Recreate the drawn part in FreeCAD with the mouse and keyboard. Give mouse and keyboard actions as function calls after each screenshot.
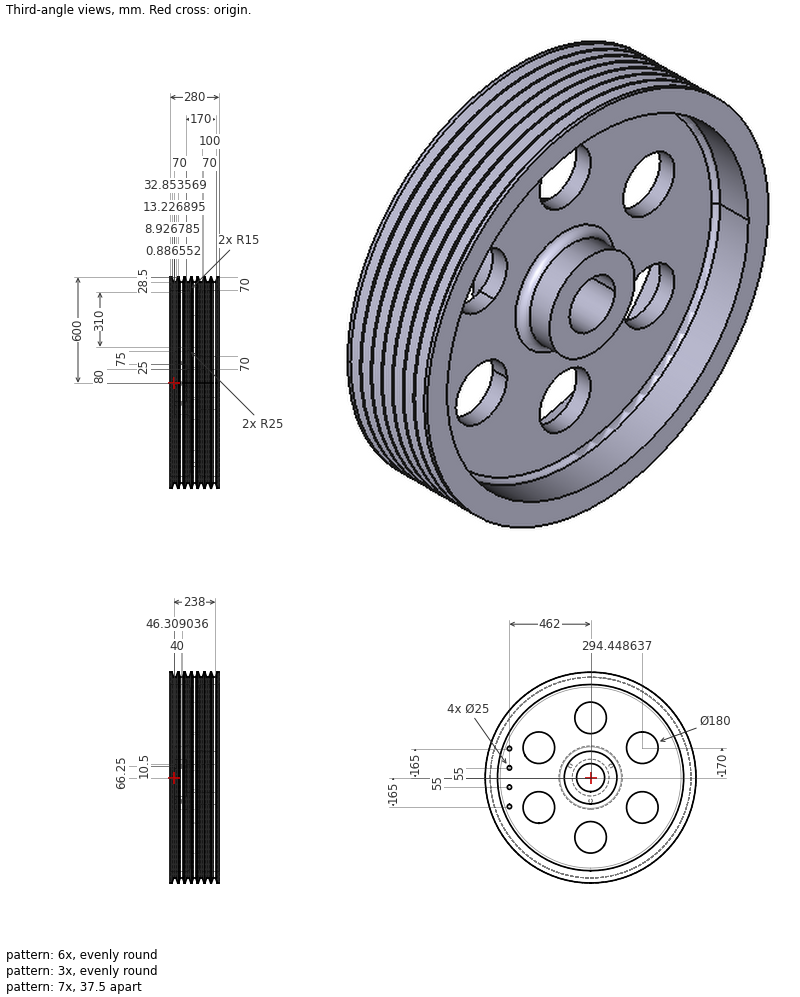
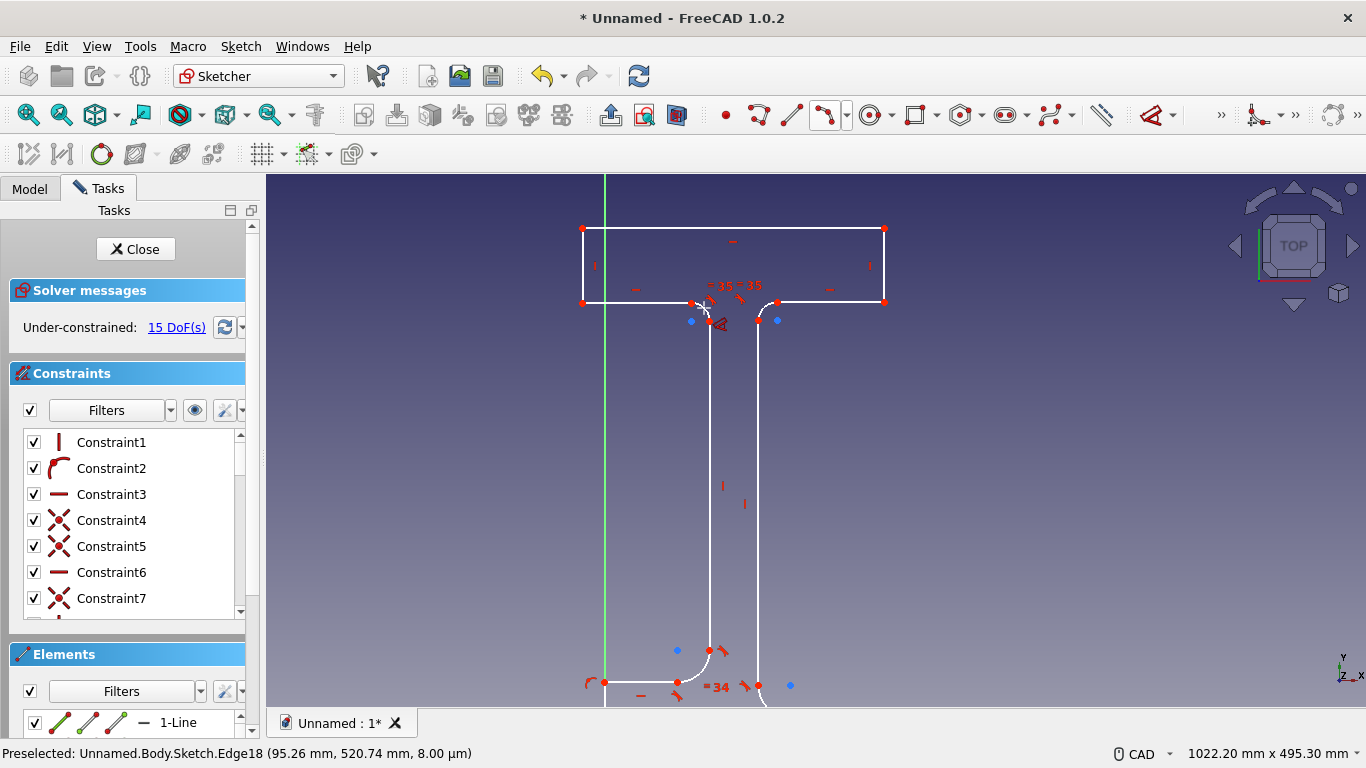
scroll(692, 679, up, 2)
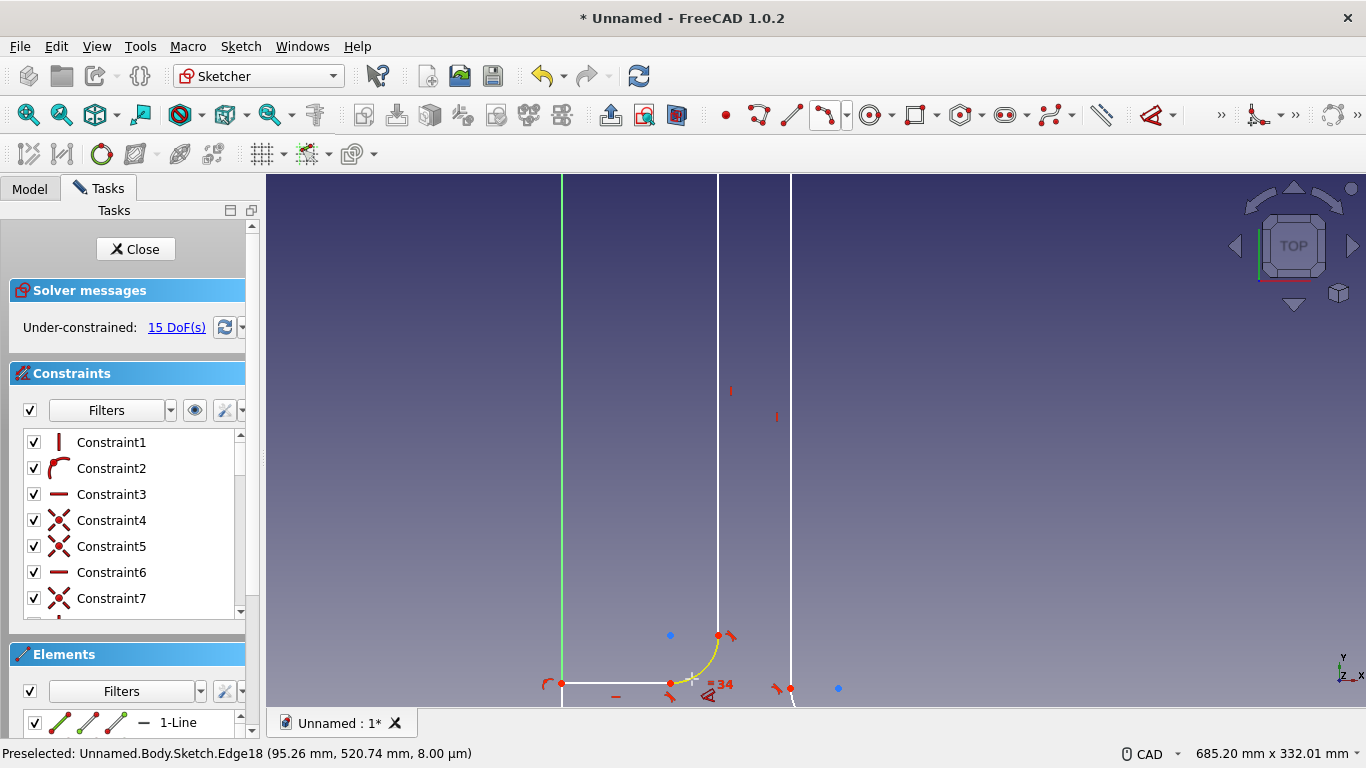
click(693, 678)
click(750, 643)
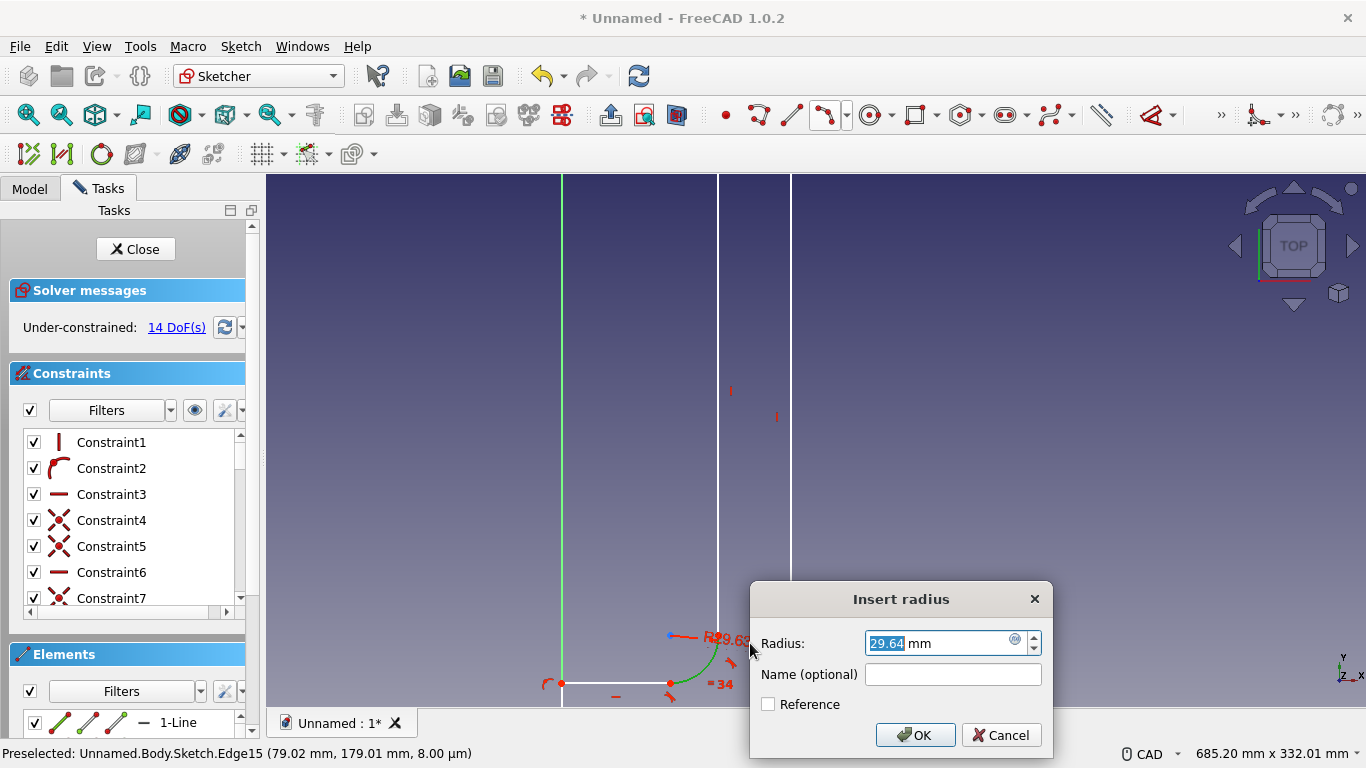
text(25)
key(Return)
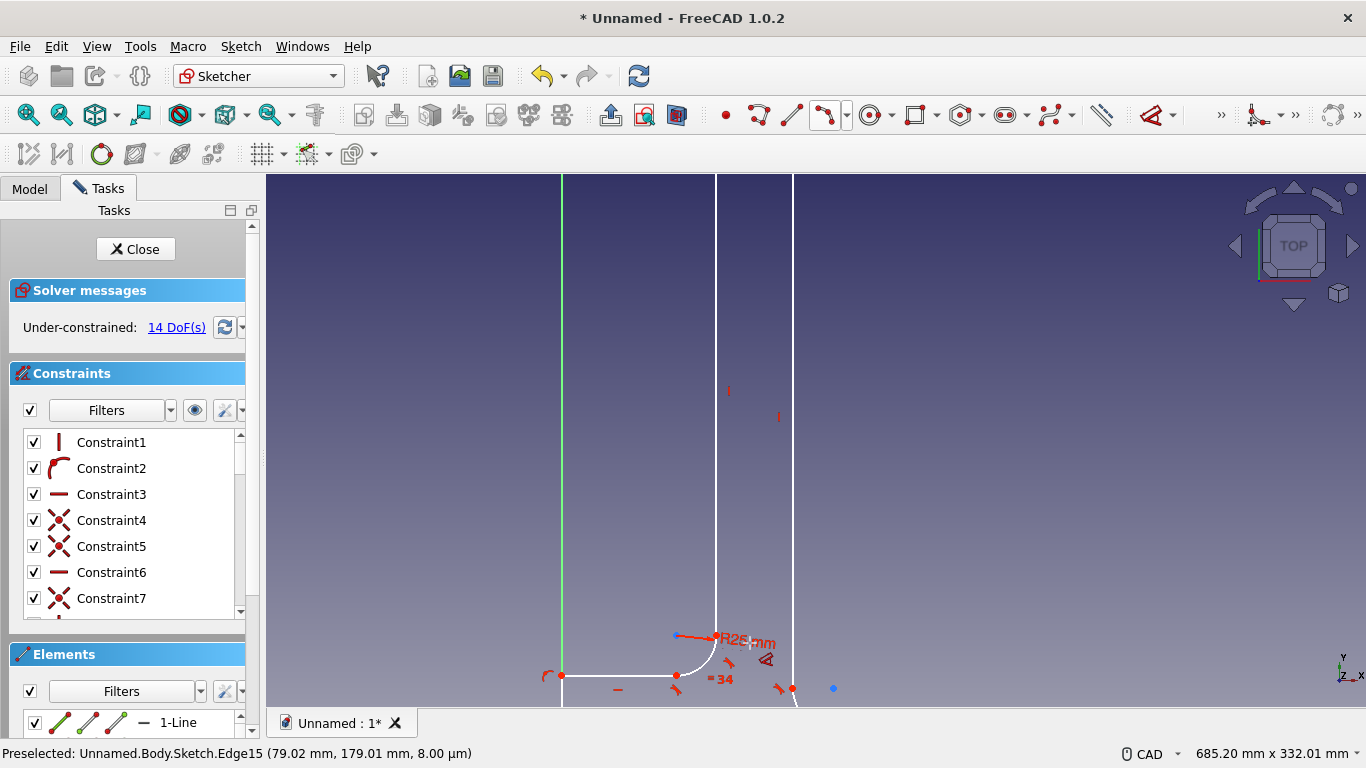
scroll(744, 414, down, 5)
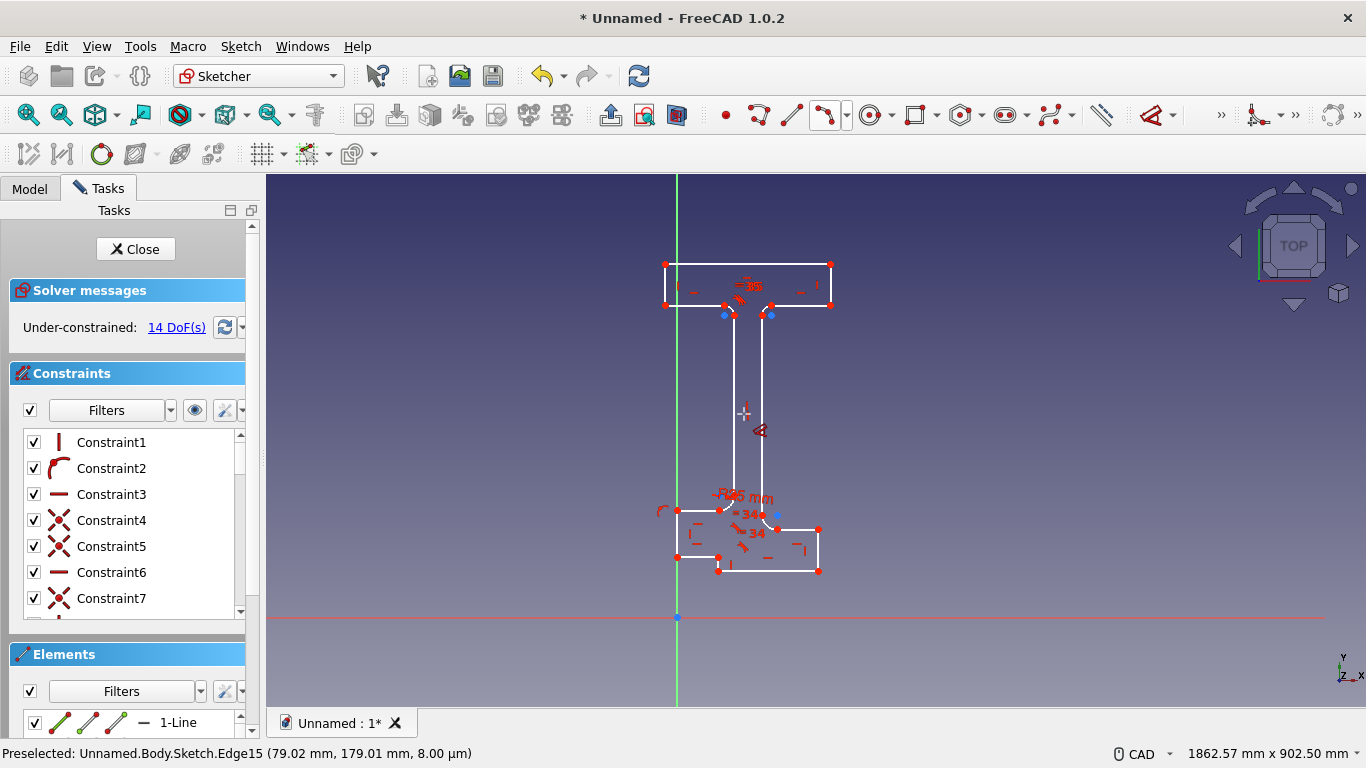
scroll(767, 307, up, 8)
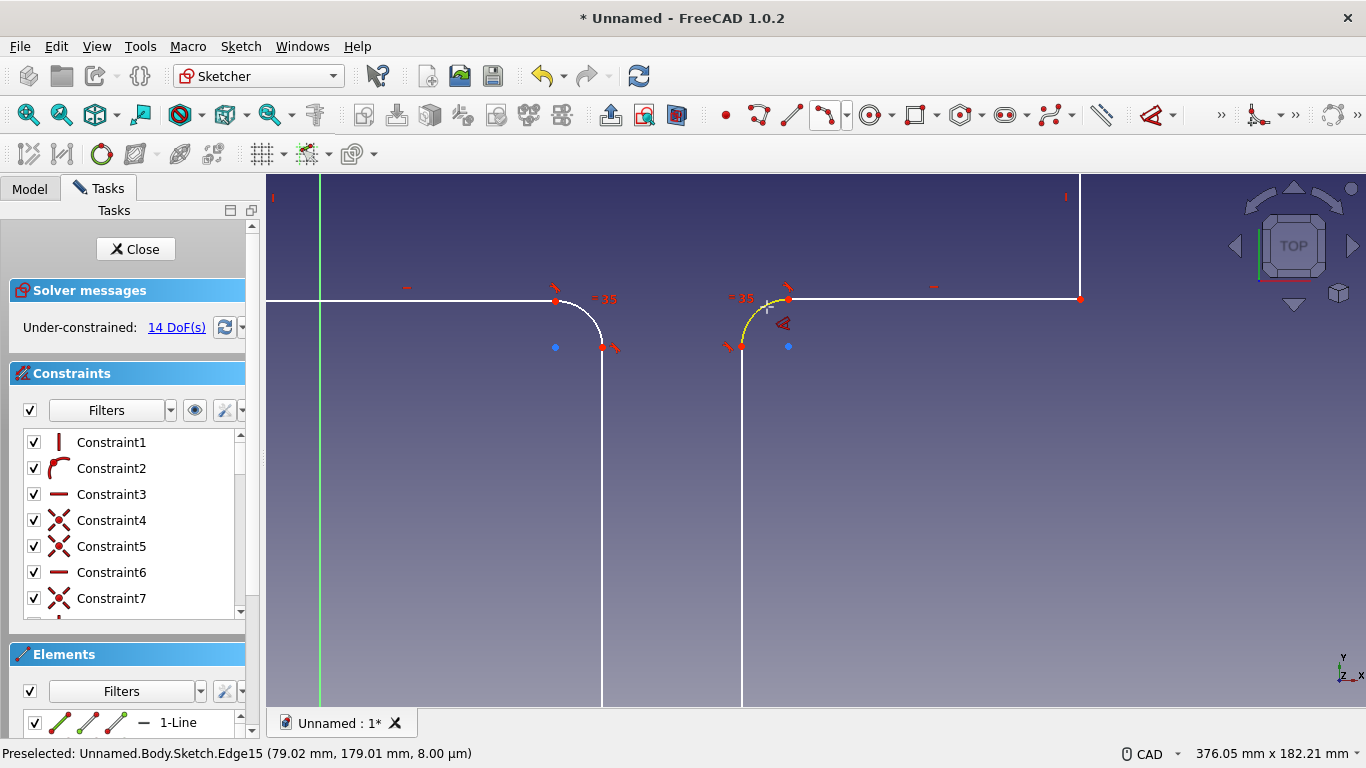
click(767, 304)
click(752, 276)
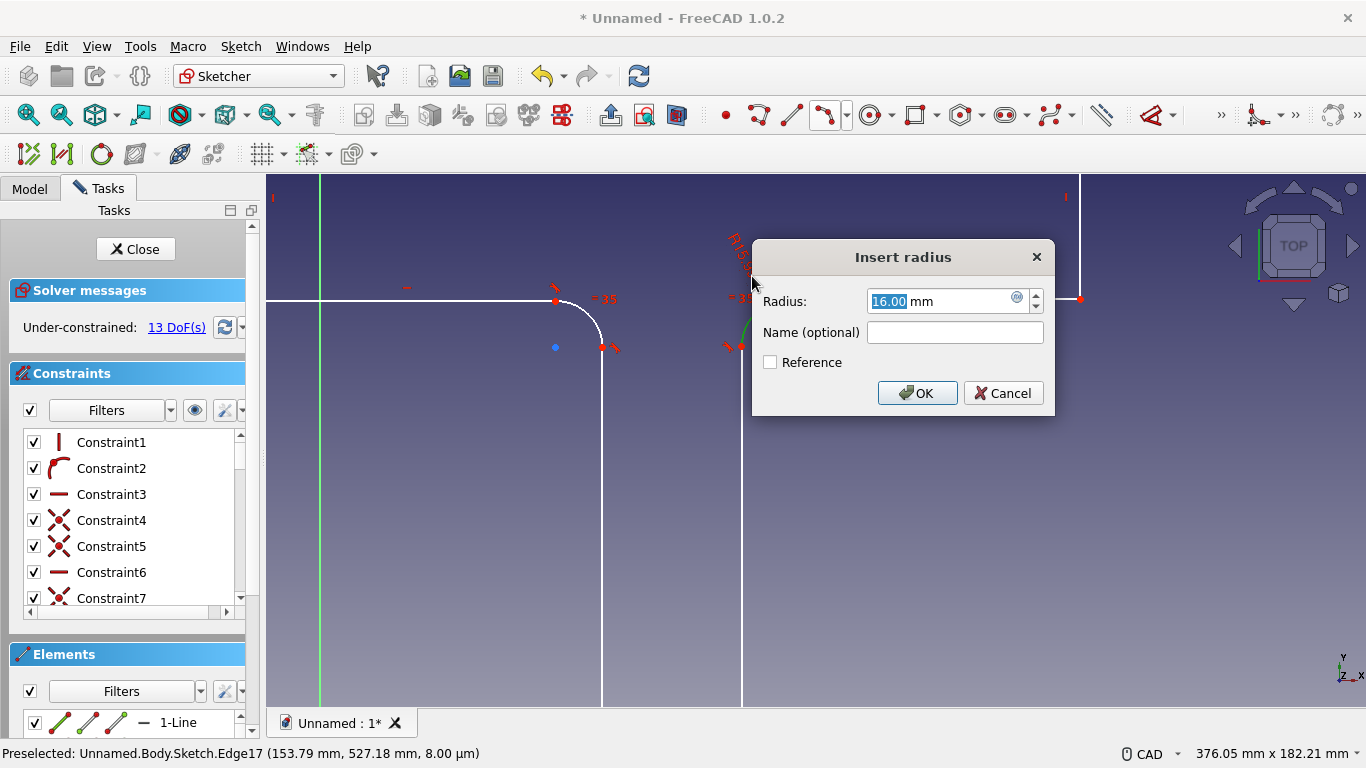
text(15)
key(Return)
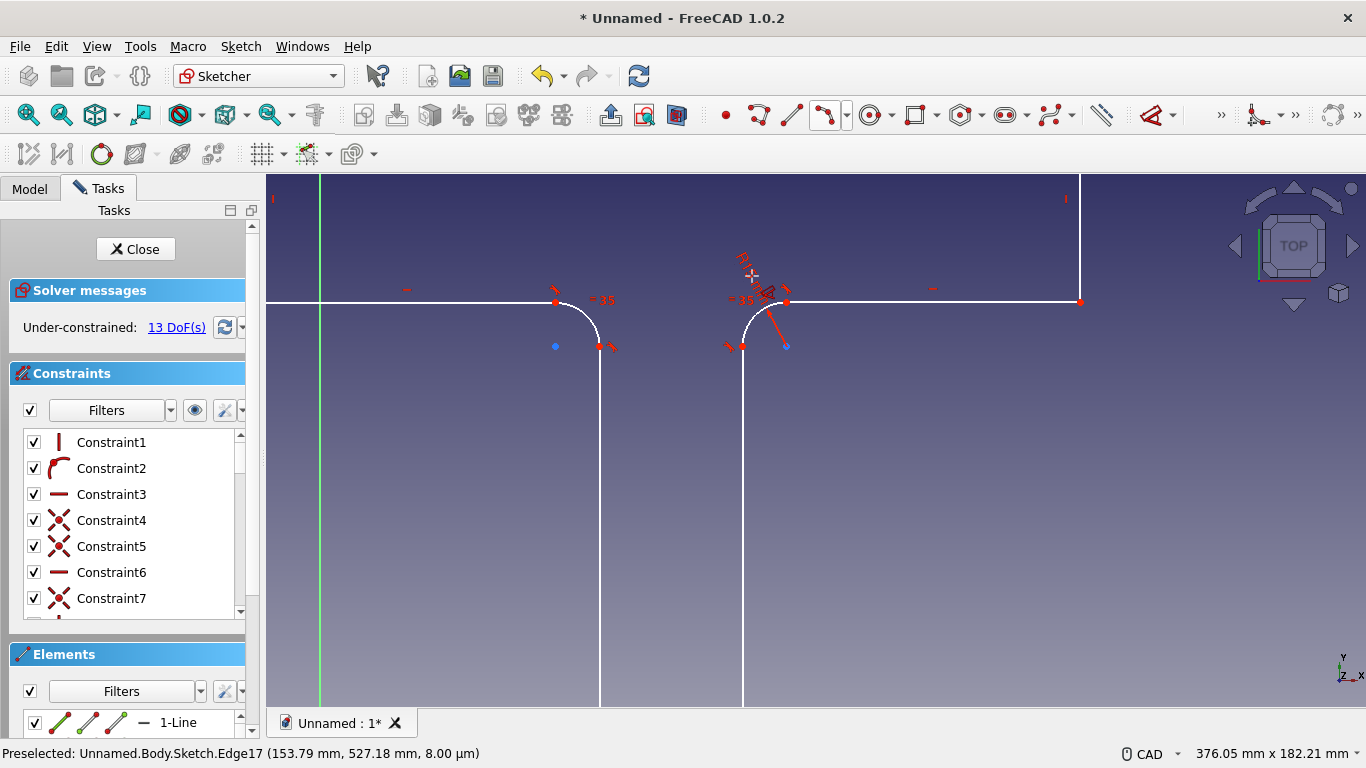
scroll(767, 307, down, 8)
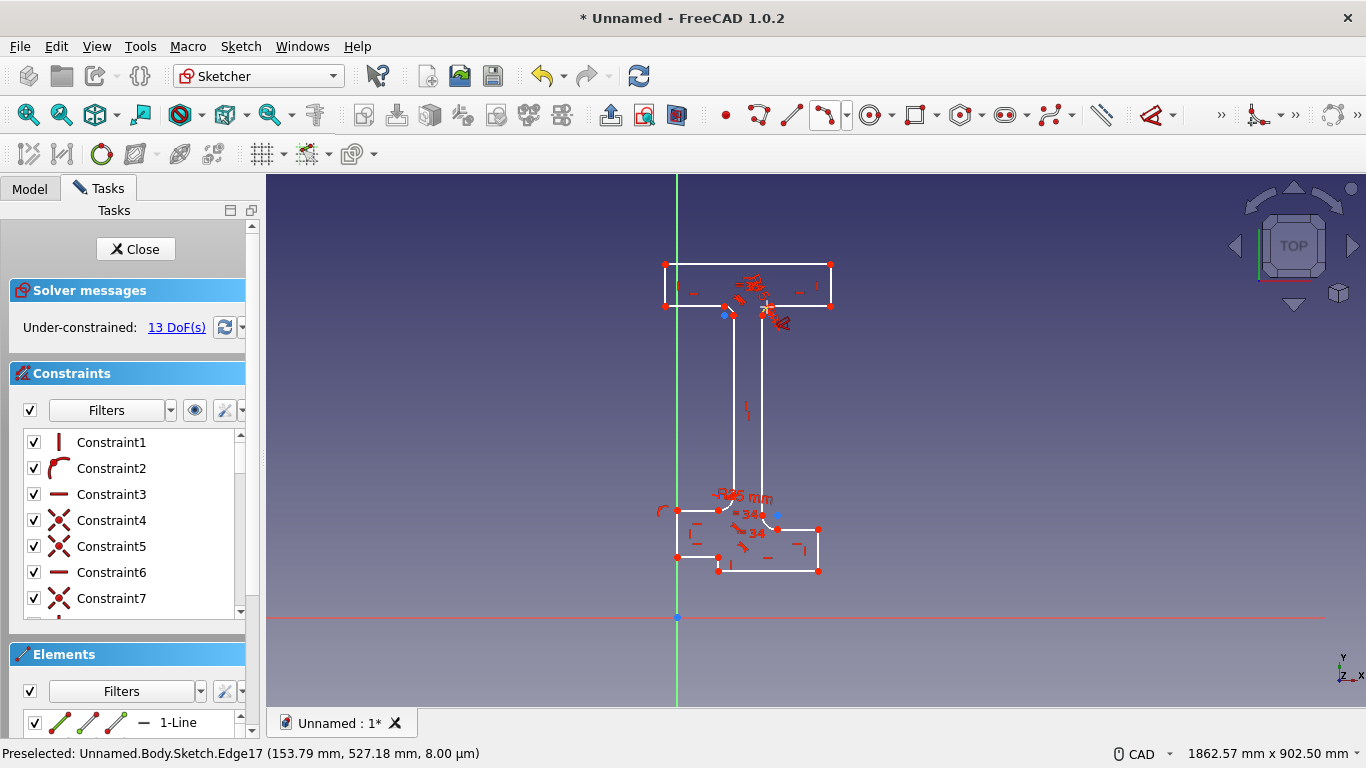
click(706, 511)
click(698, 477)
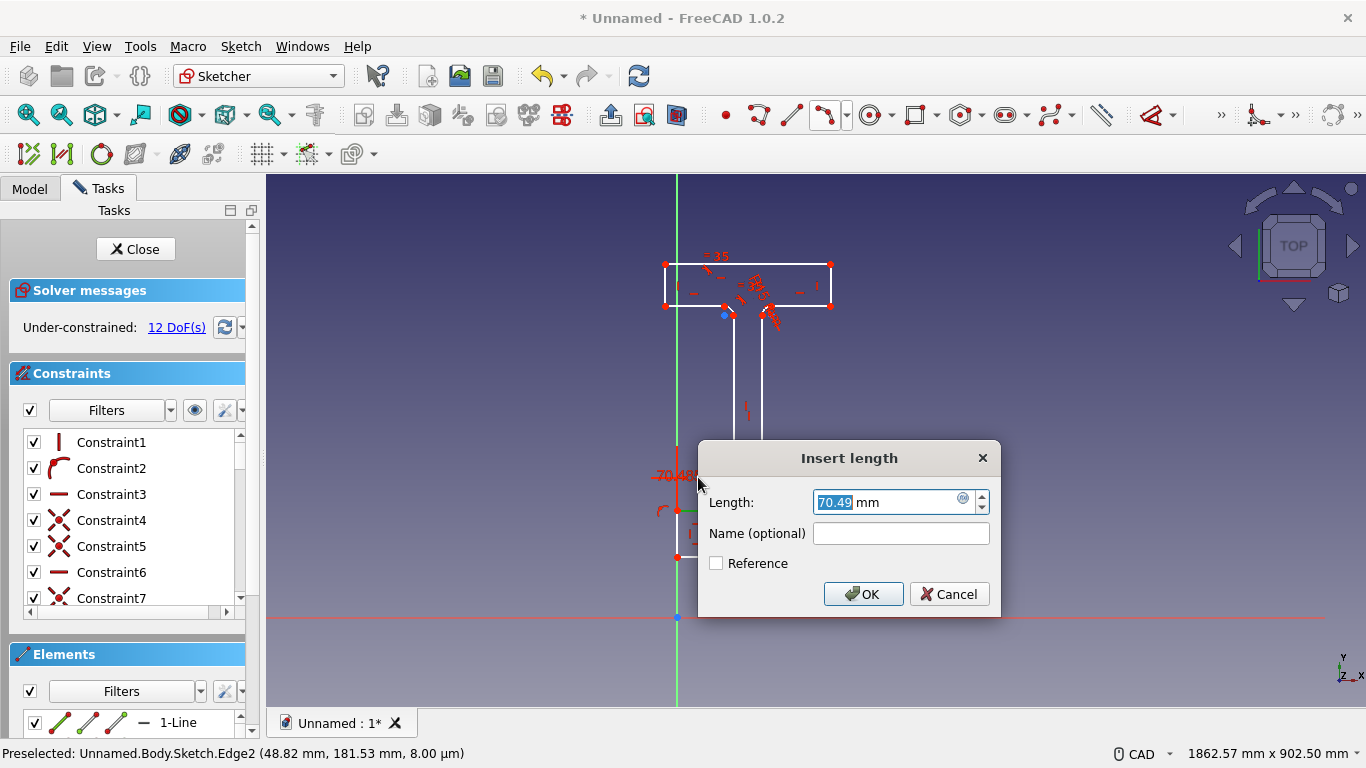
text(70)
key(Return)